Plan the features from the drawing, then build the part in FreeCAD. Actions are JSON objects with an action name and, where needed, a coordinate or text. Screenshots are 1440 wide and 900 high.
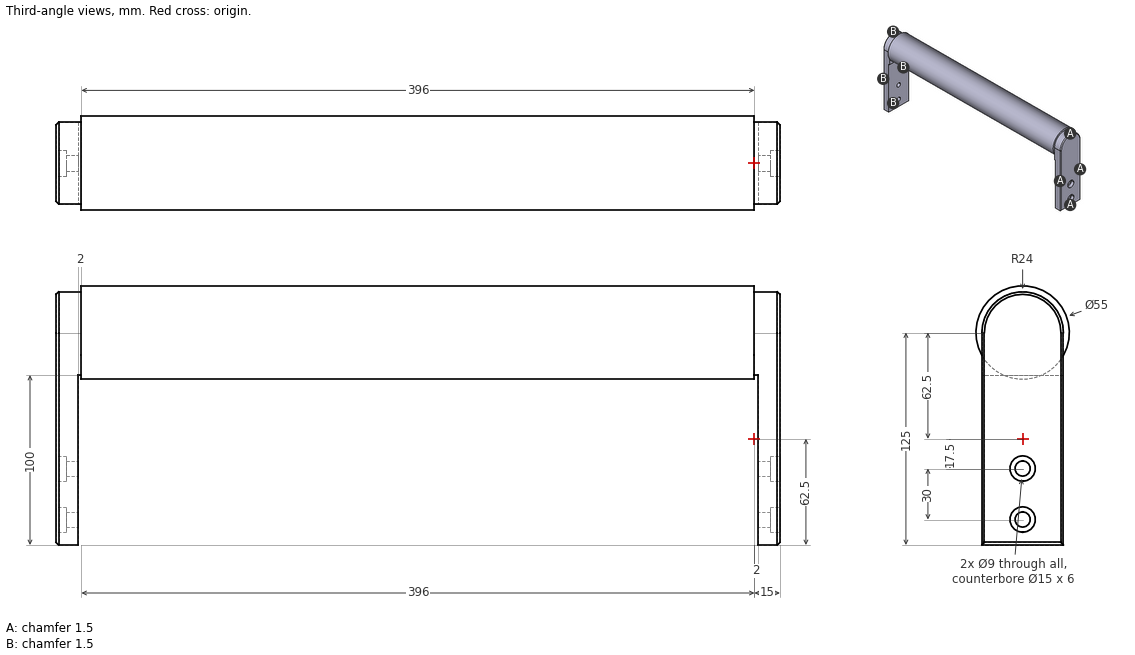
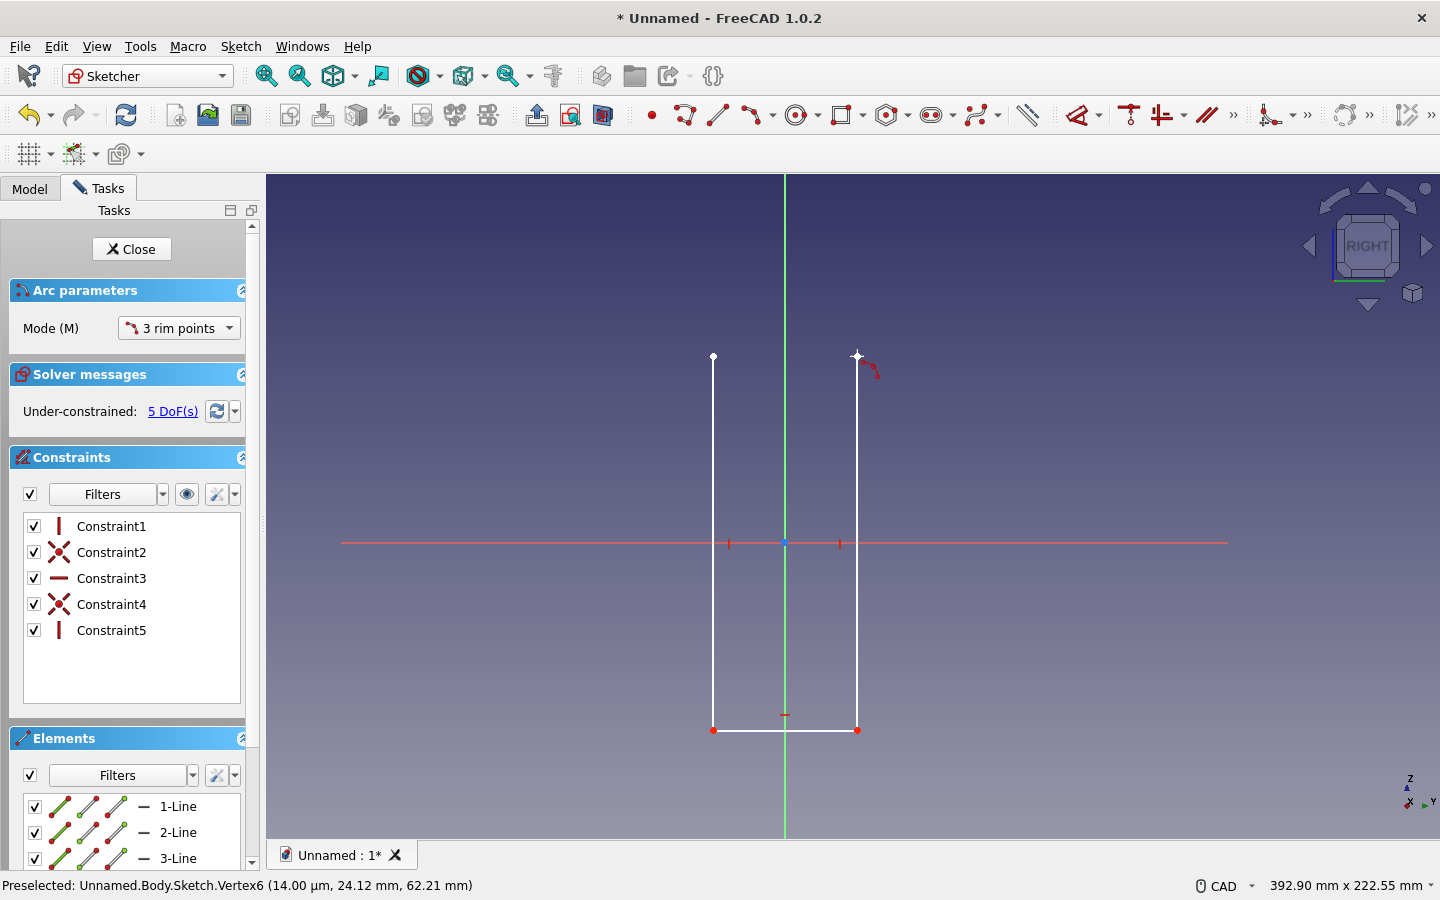
{"action": "left_click", "coordinate": [857, 357]}
{"action": "left_click", "coordinate": [713, 357]}
{"action": "left_click", "coordinate": [807, 288]}
{"action": "key", "text": "Escape"}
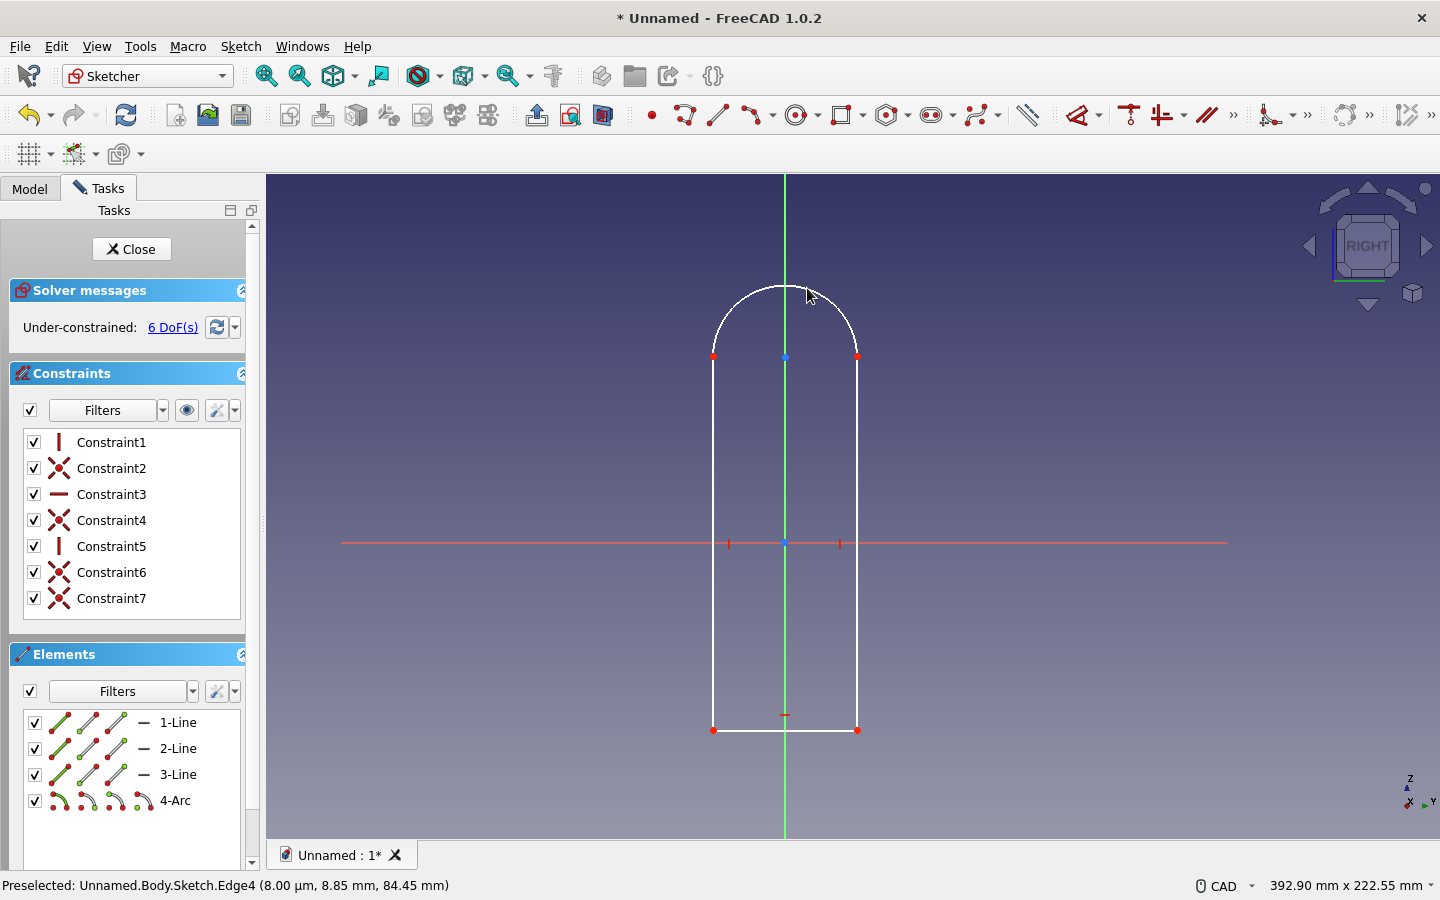
{"action": "left_click", "coordinate": [713, 469]}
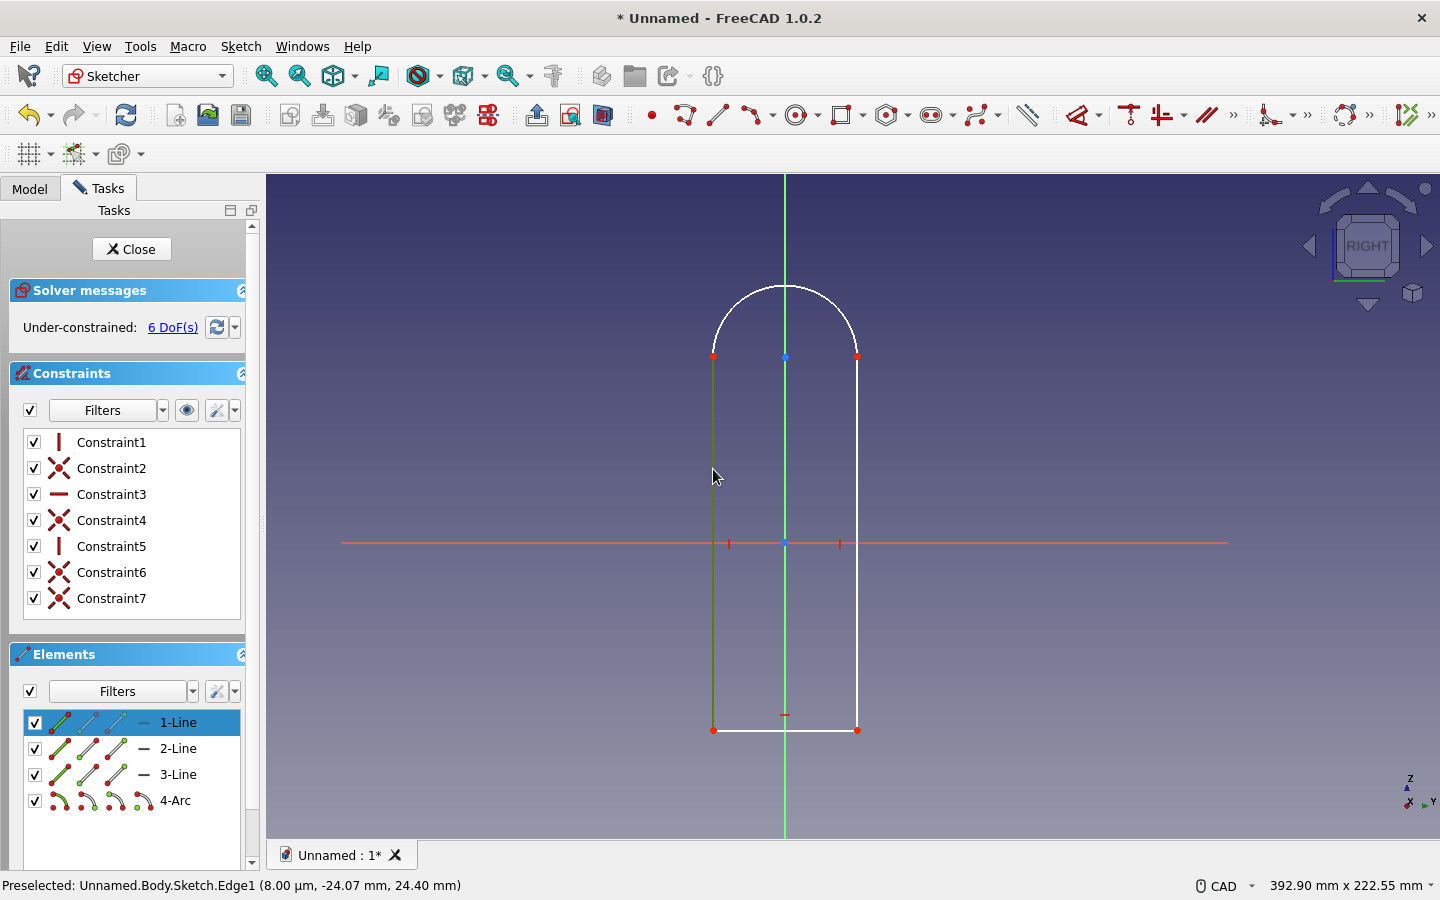
{"action": "left_click", "coordinate": [827, 299]}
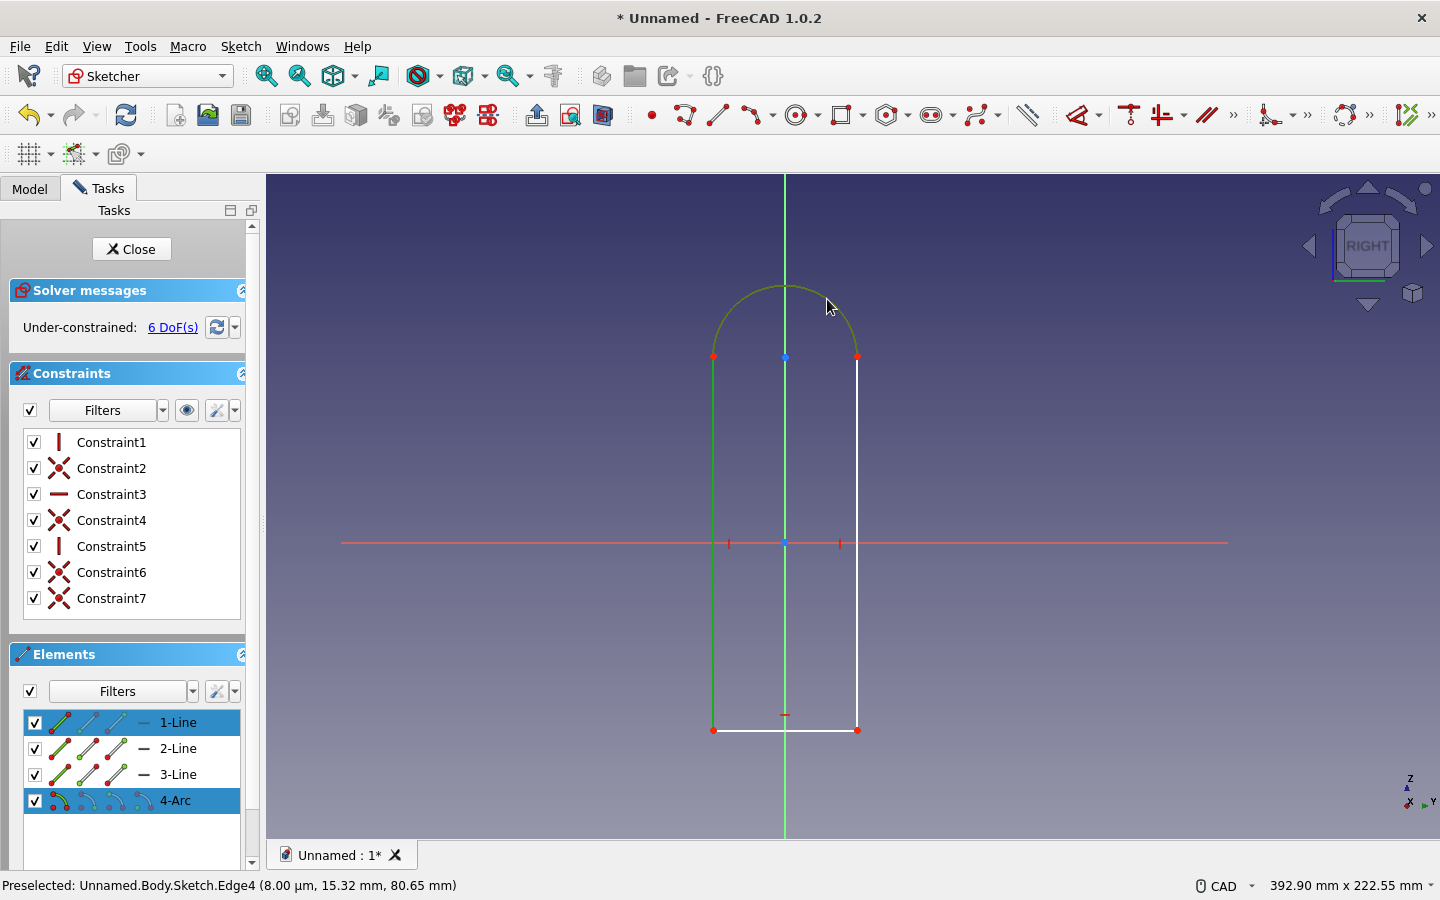
{"action": "key", "text": "t"}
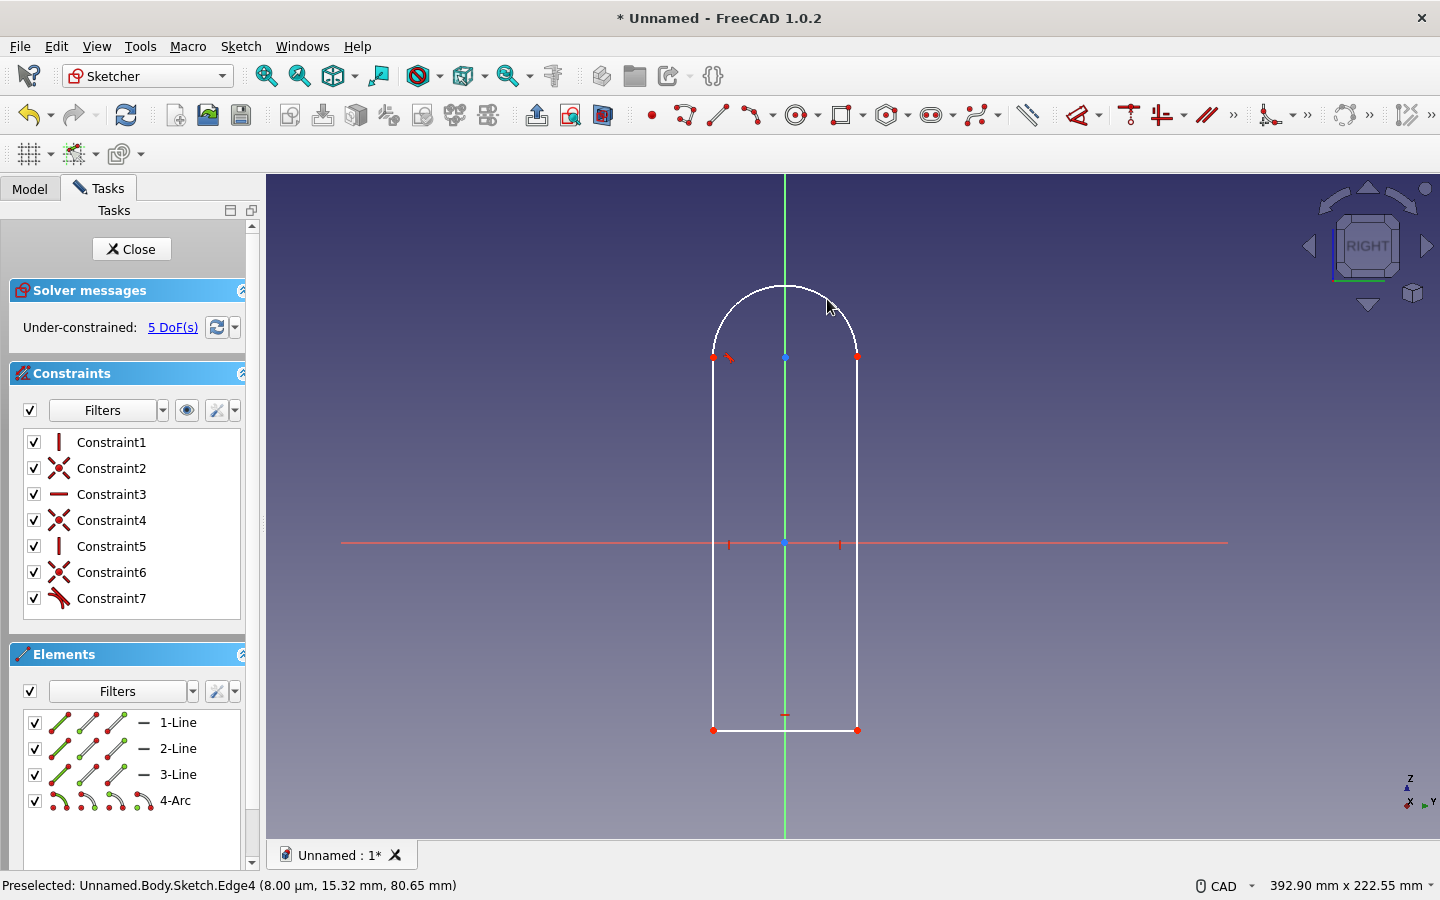
{"action": "left_click", "coordinate": [857, 619]}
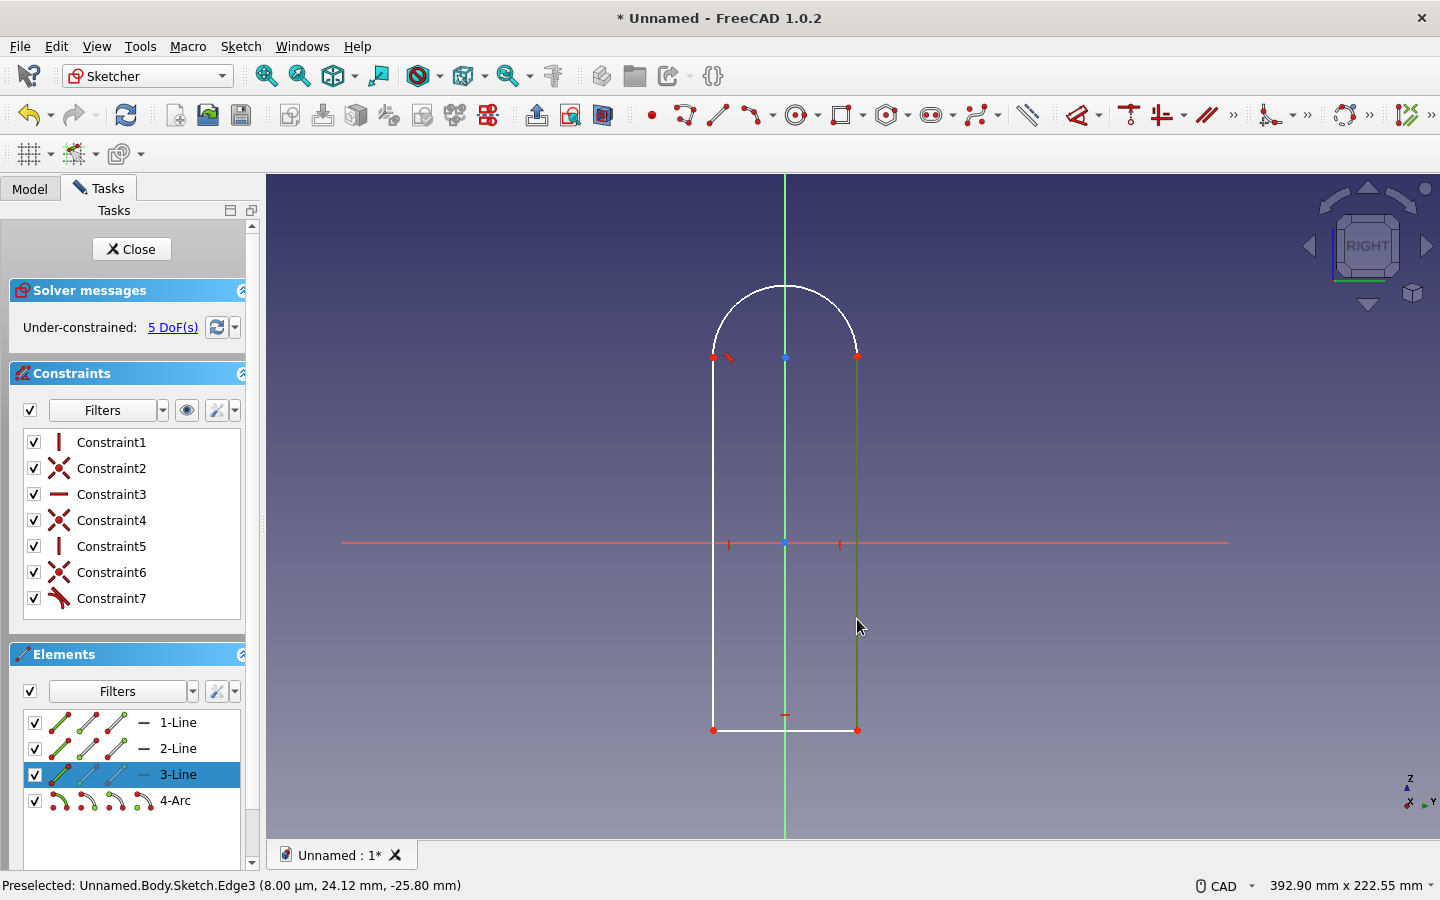
{"action": "left_click", "coordinate": [827, 299]}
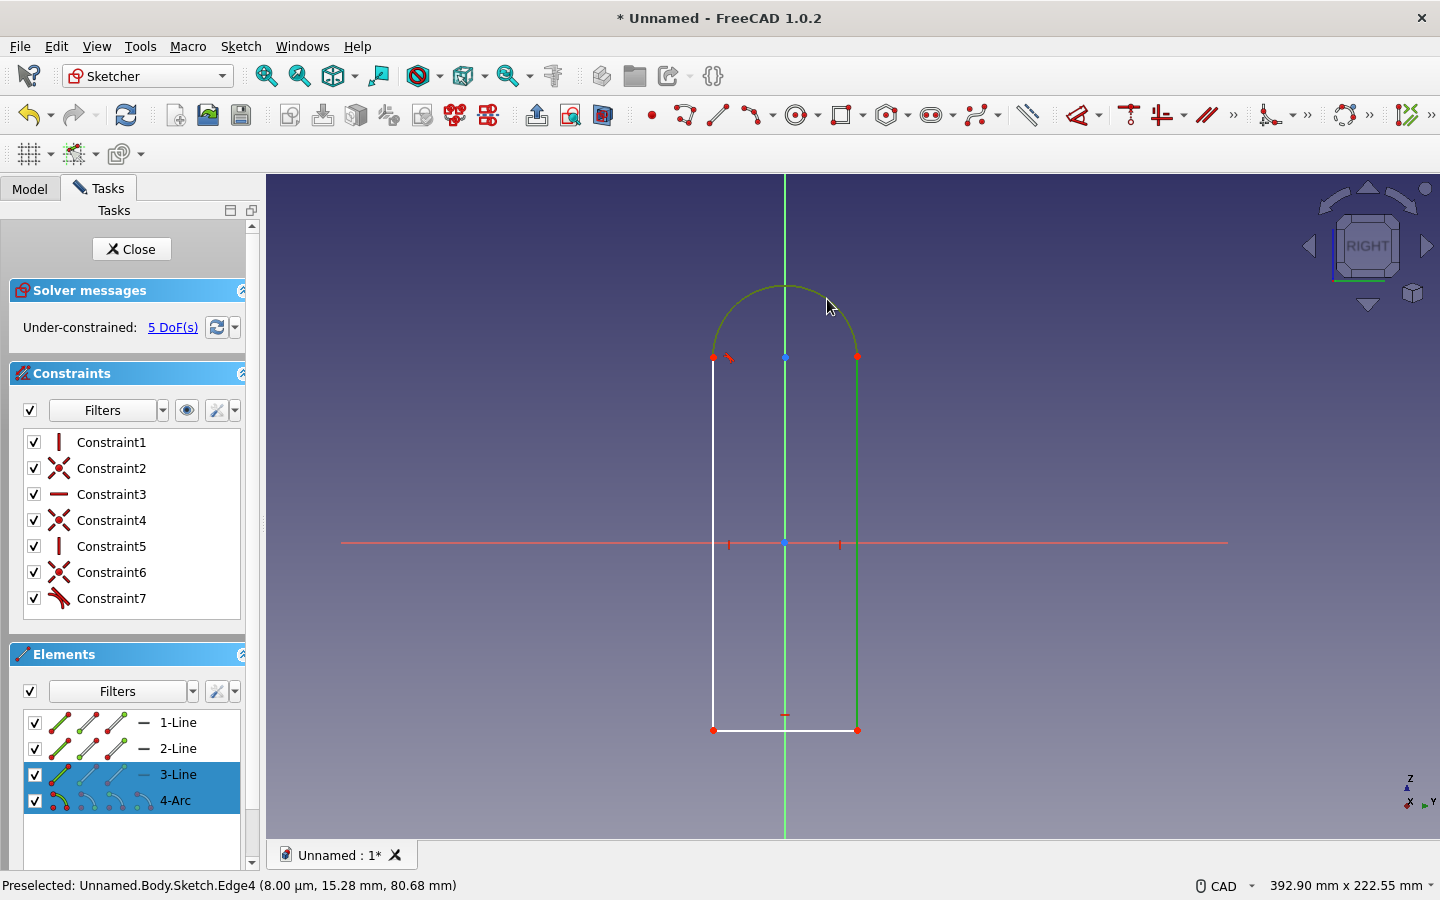
{"action": "key", "text": "t"}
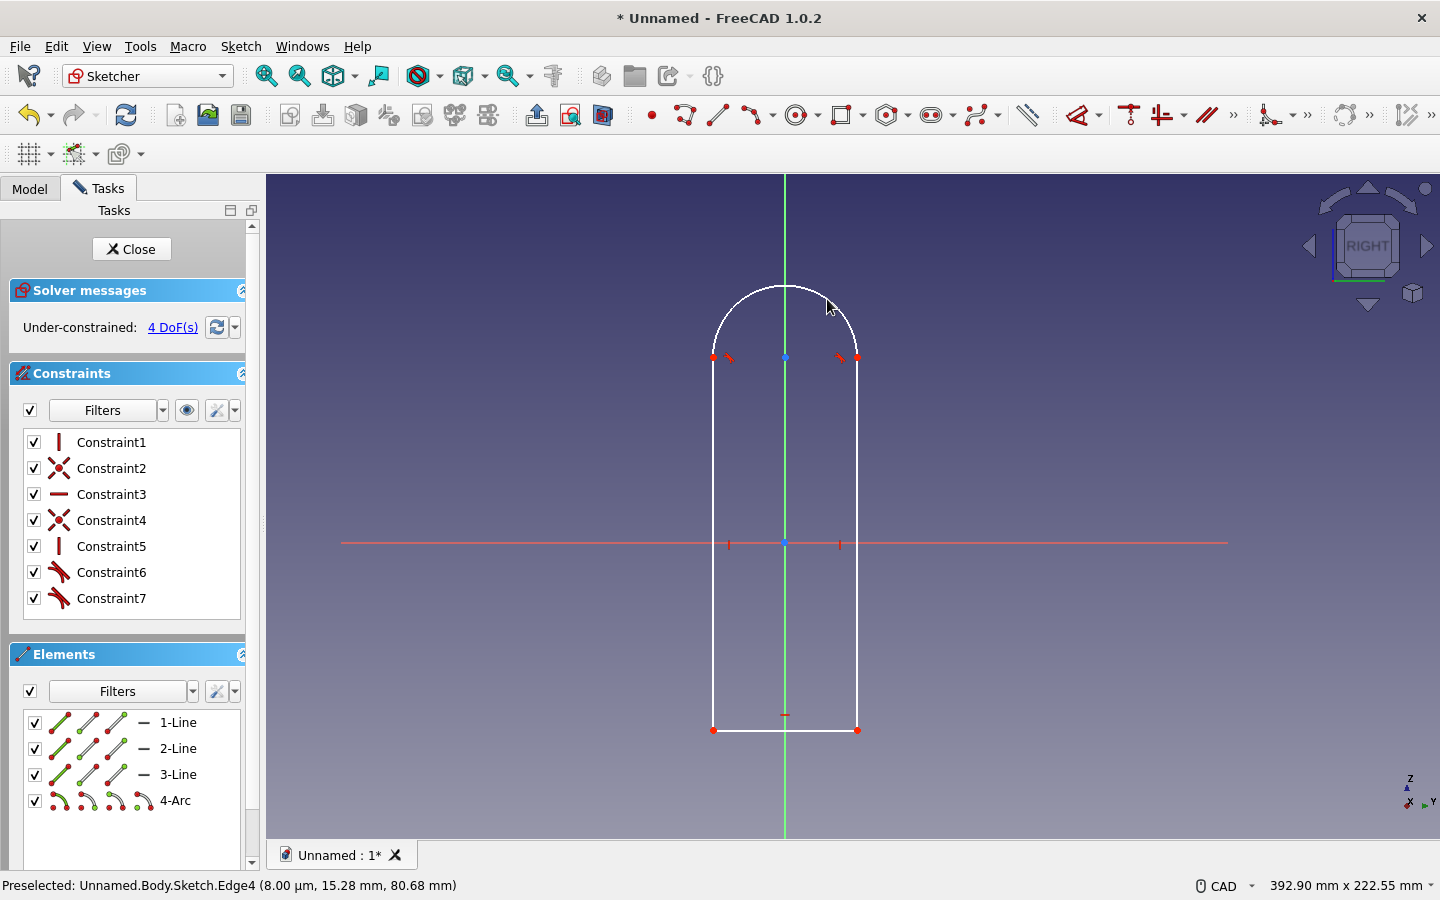
{"action": "left_click", "coordinate": [785, 358]}